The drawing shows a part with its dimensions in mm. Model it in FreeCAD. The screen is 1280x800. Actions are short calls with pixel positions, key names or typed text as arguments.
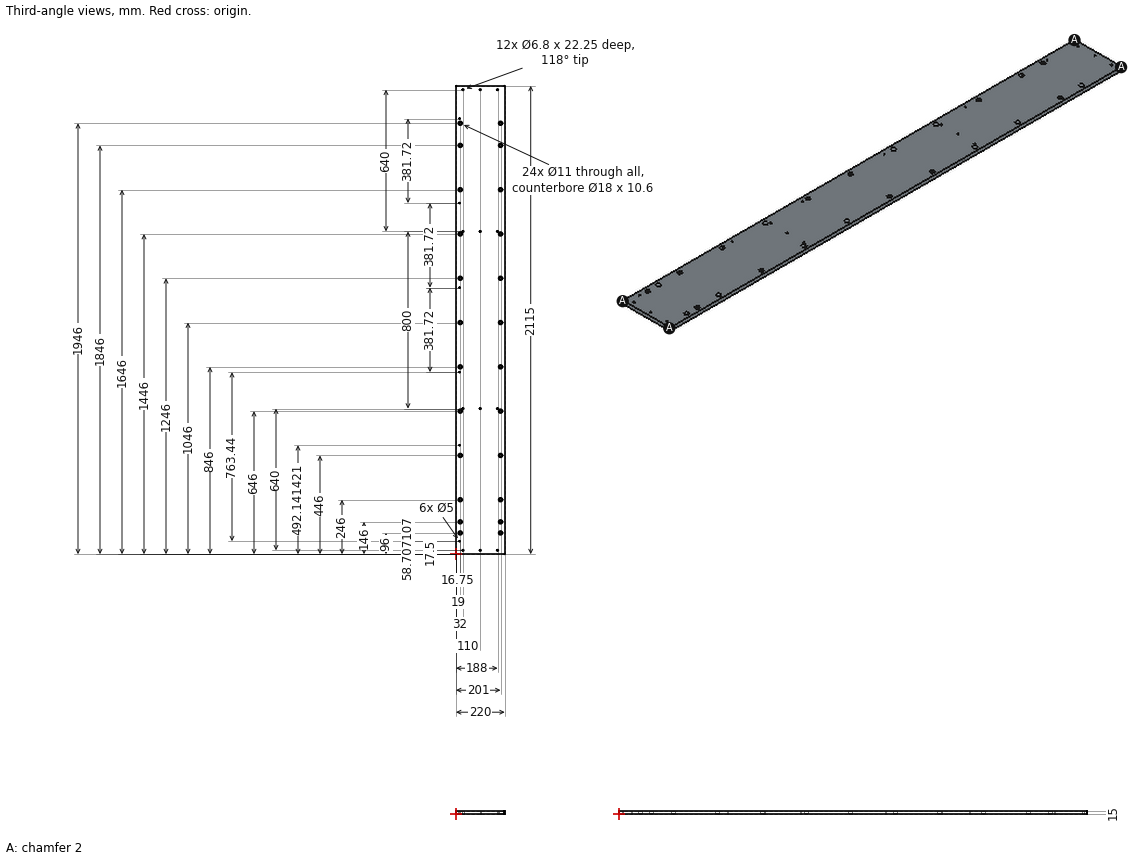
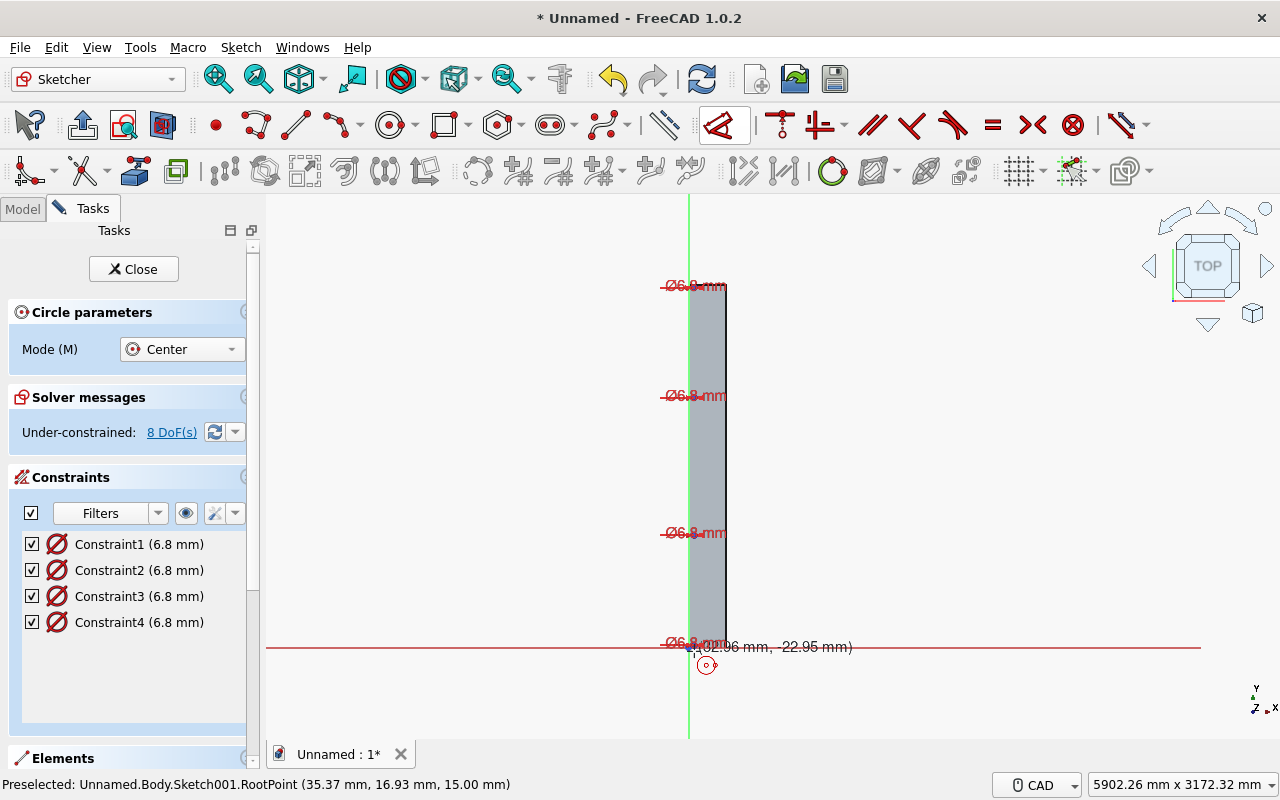
scroll(708, 288, up, 19)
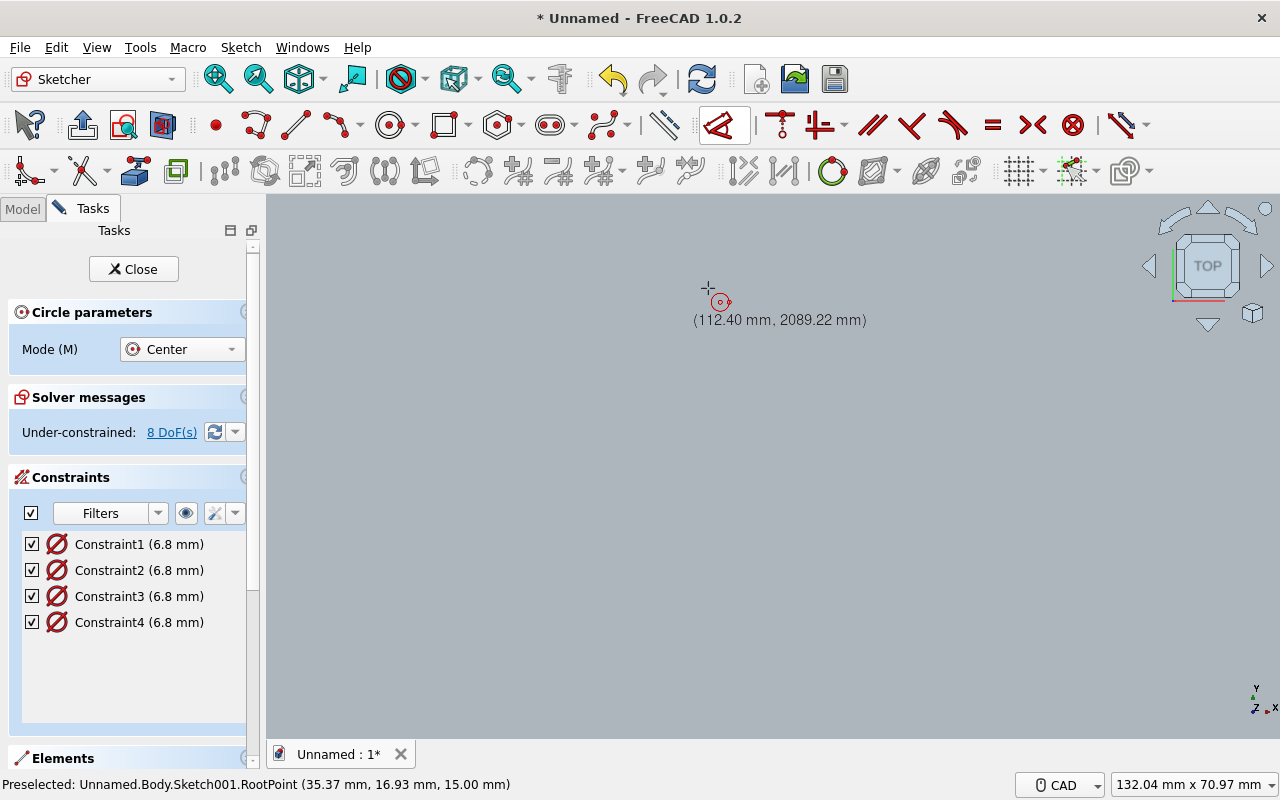
scroll(704, 466, down, 15)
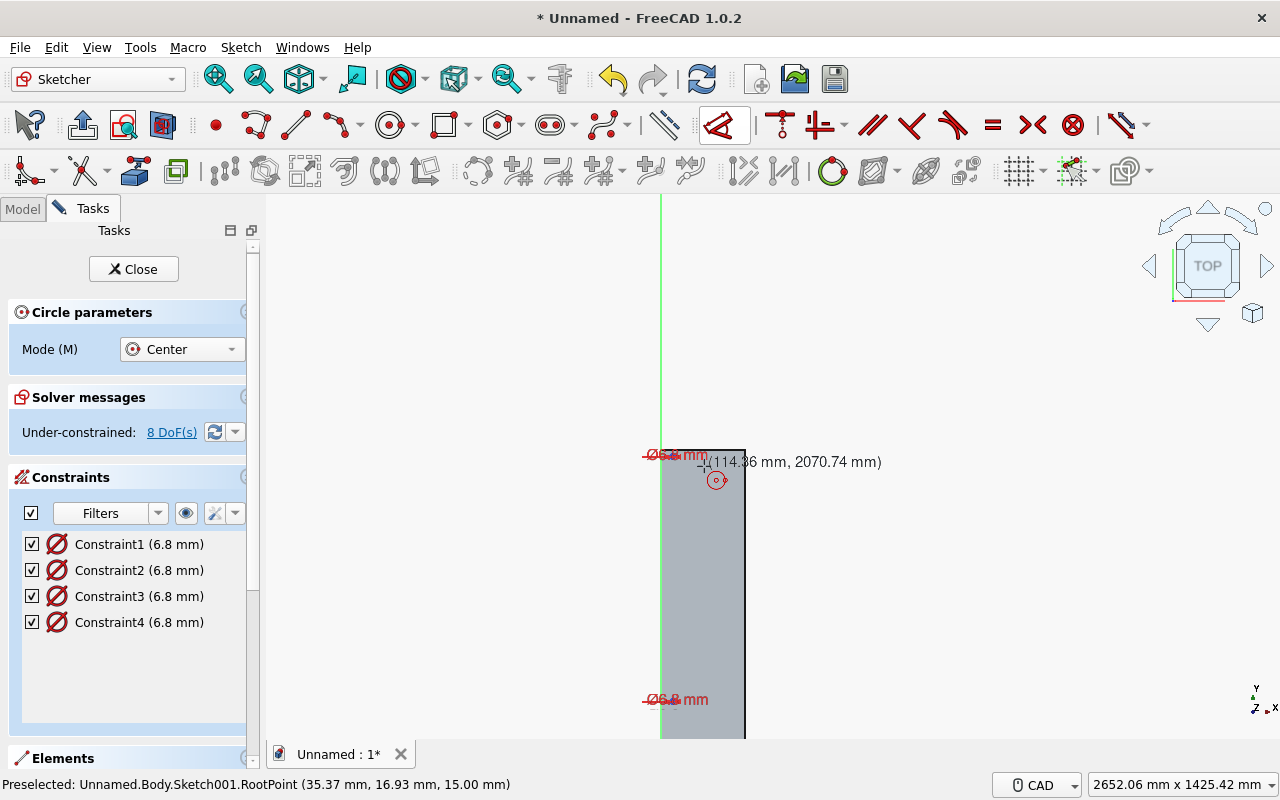
scroll(709, 239, down, 5)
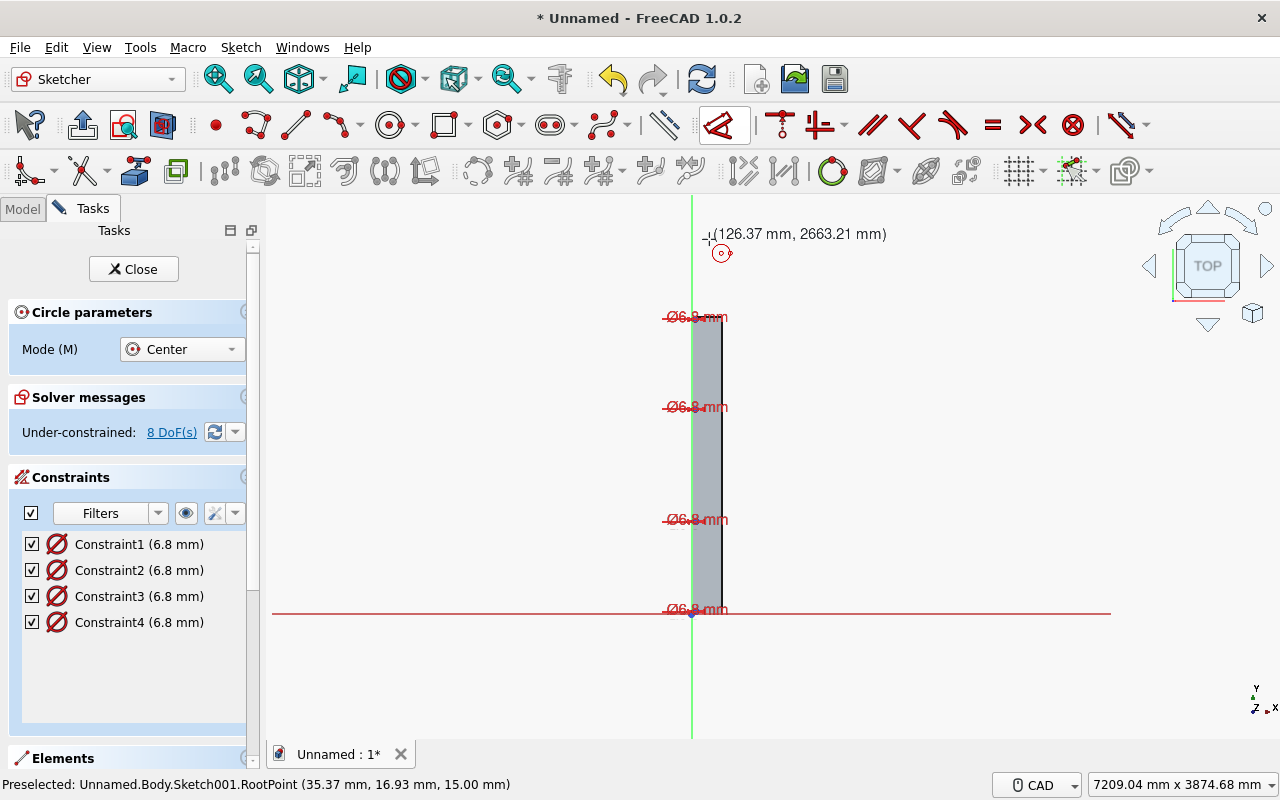
scroll(707, 319, up, 3)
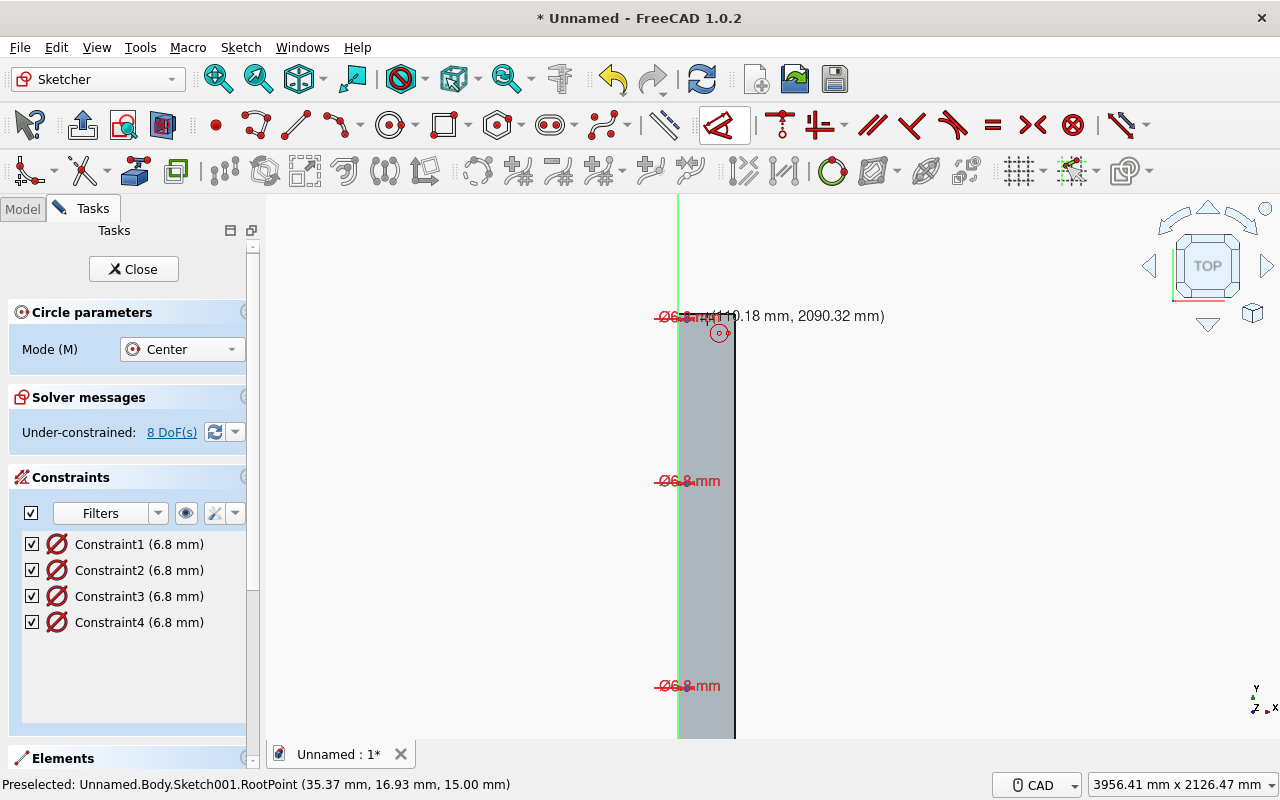
click(707, 319)
move(707, 318)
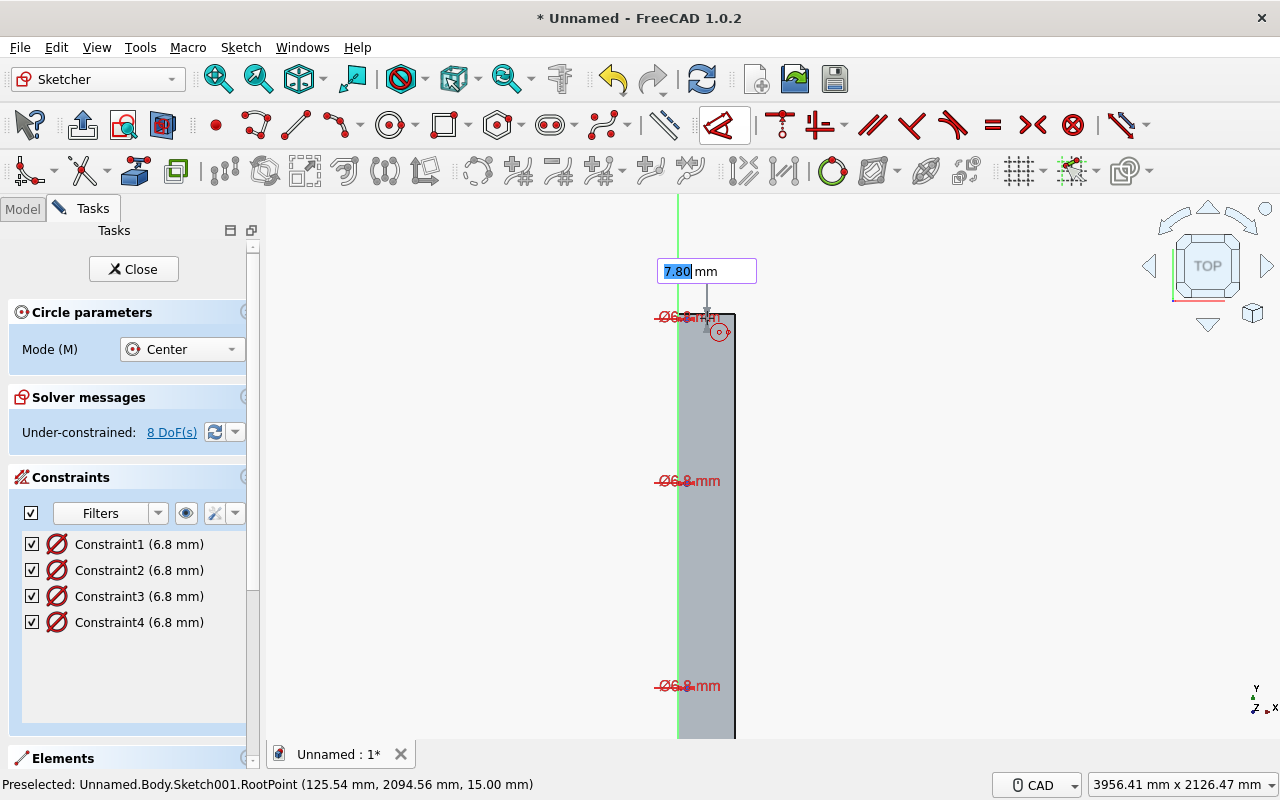
text(6.8)
key(Return)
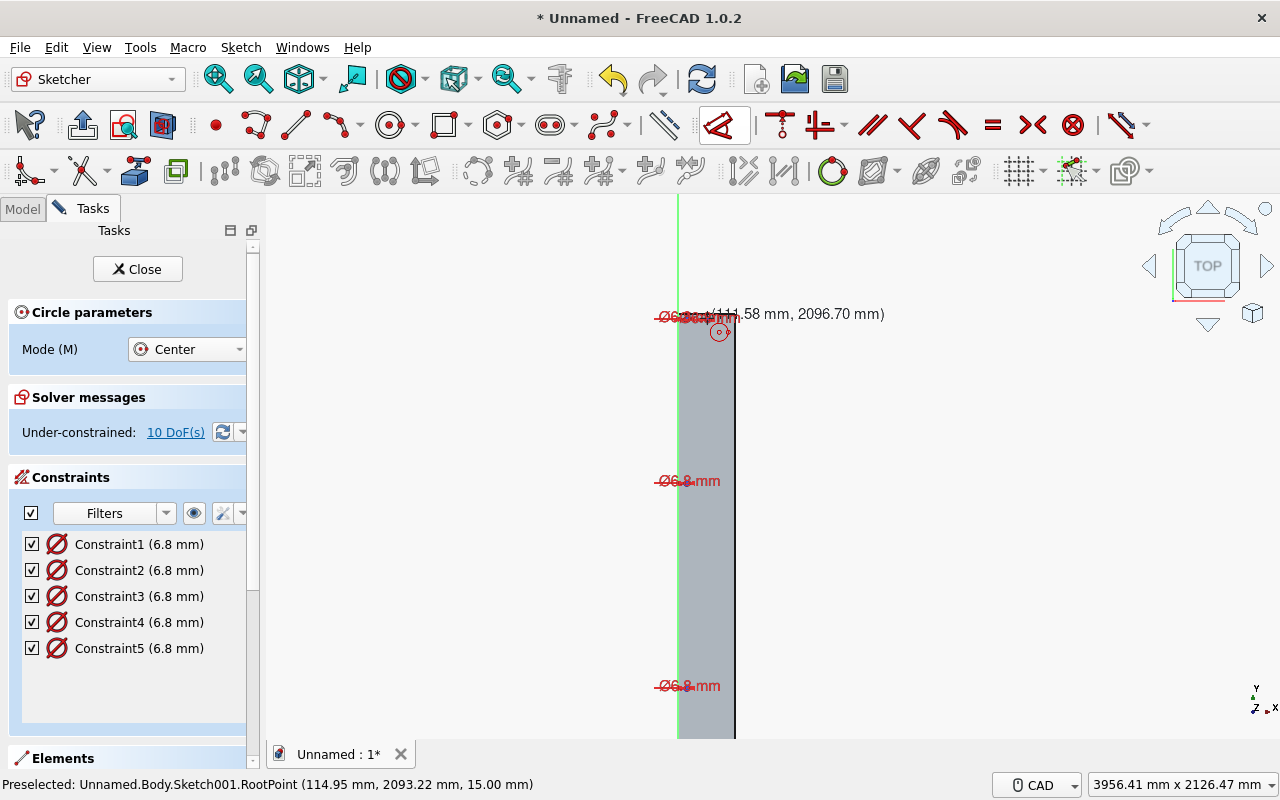
scroll(707, 483, up, 17)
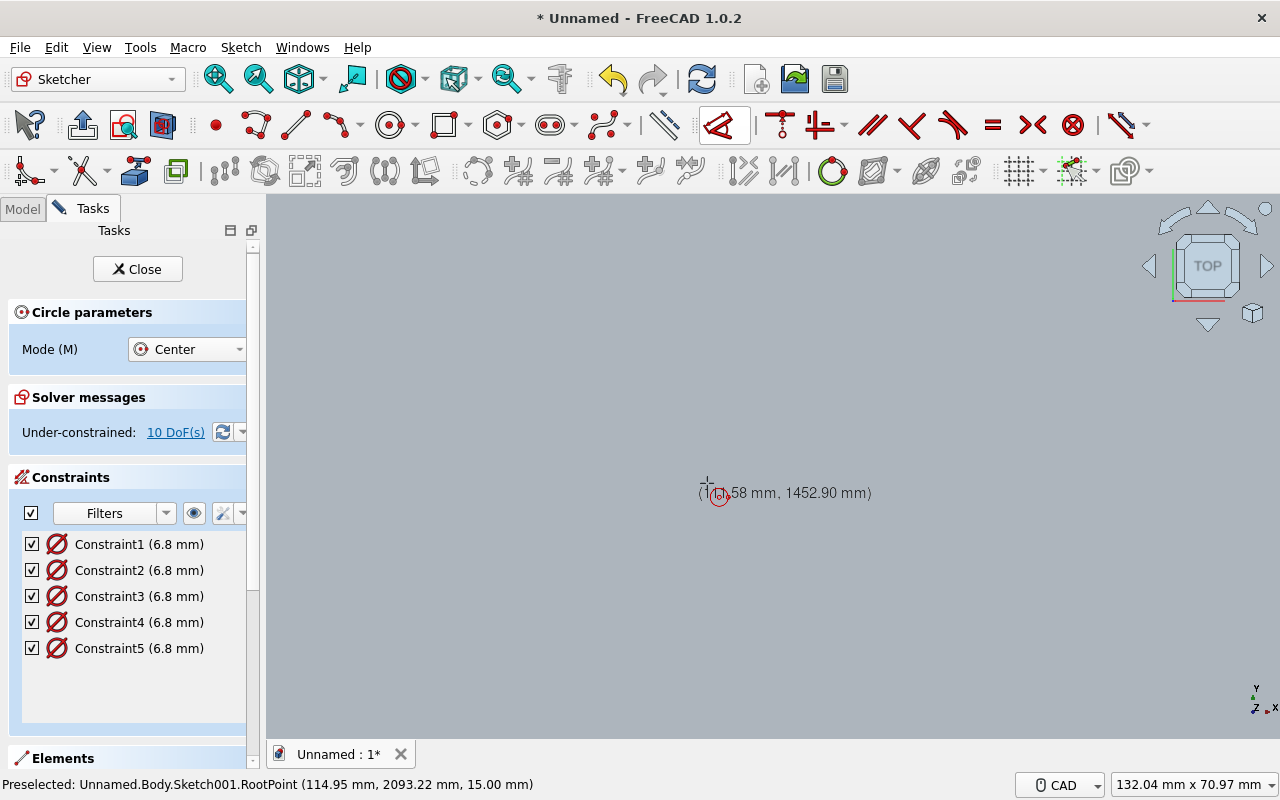
scroll(704, 466, down, 15)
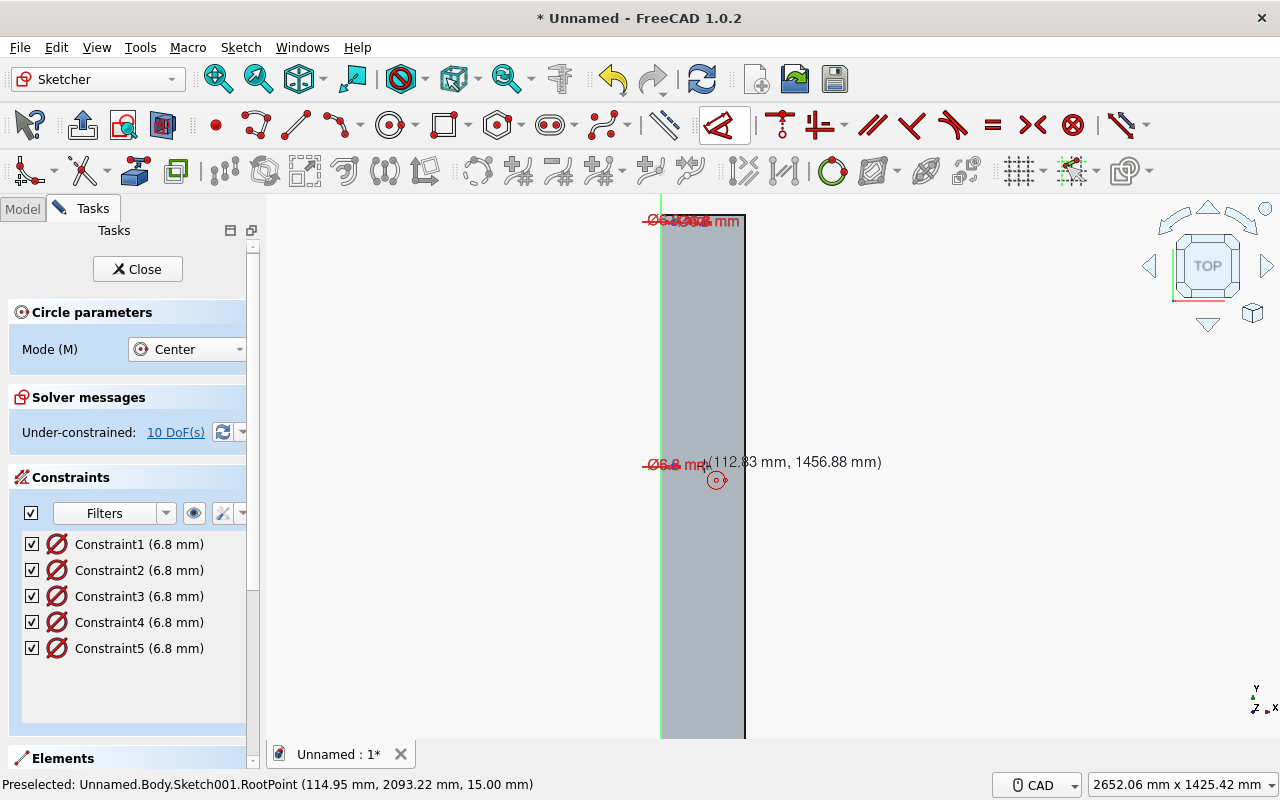
scroll(710, 340, down, 4)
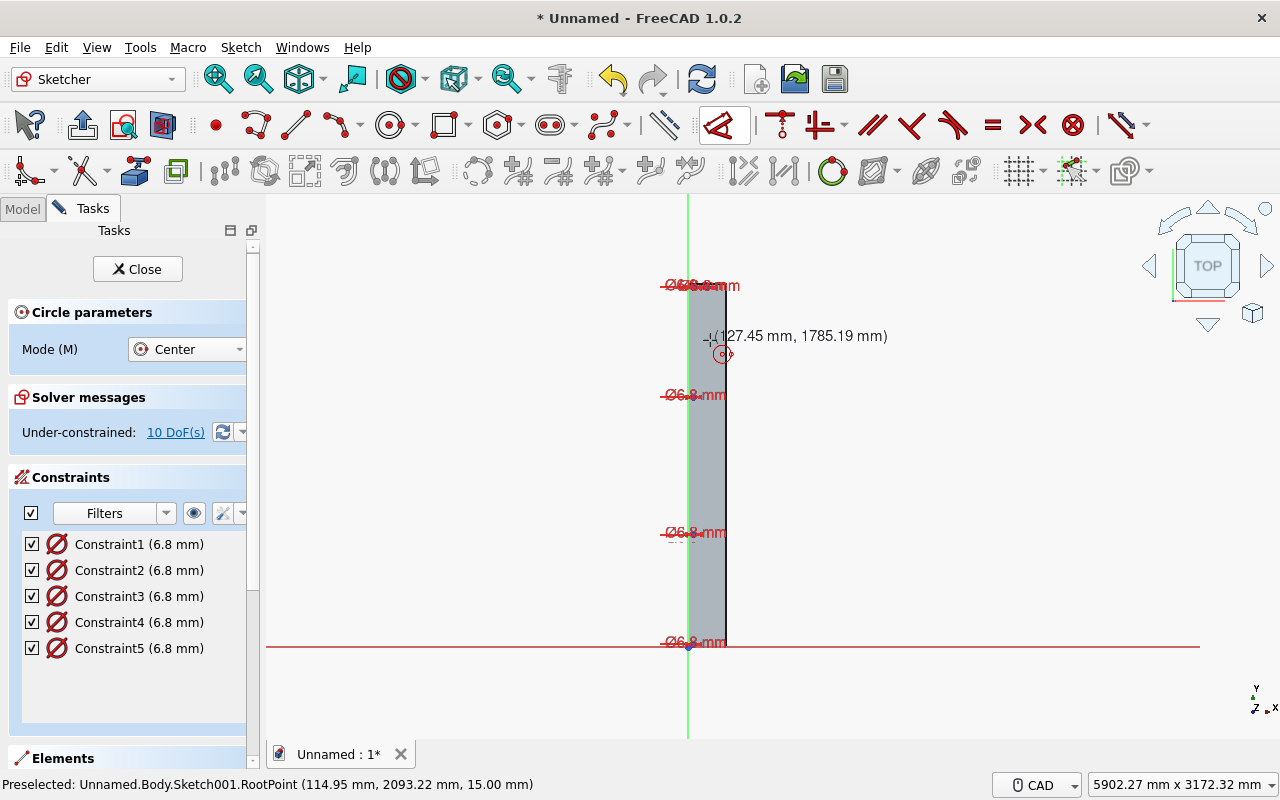
scroll(707, 397, up, 2)